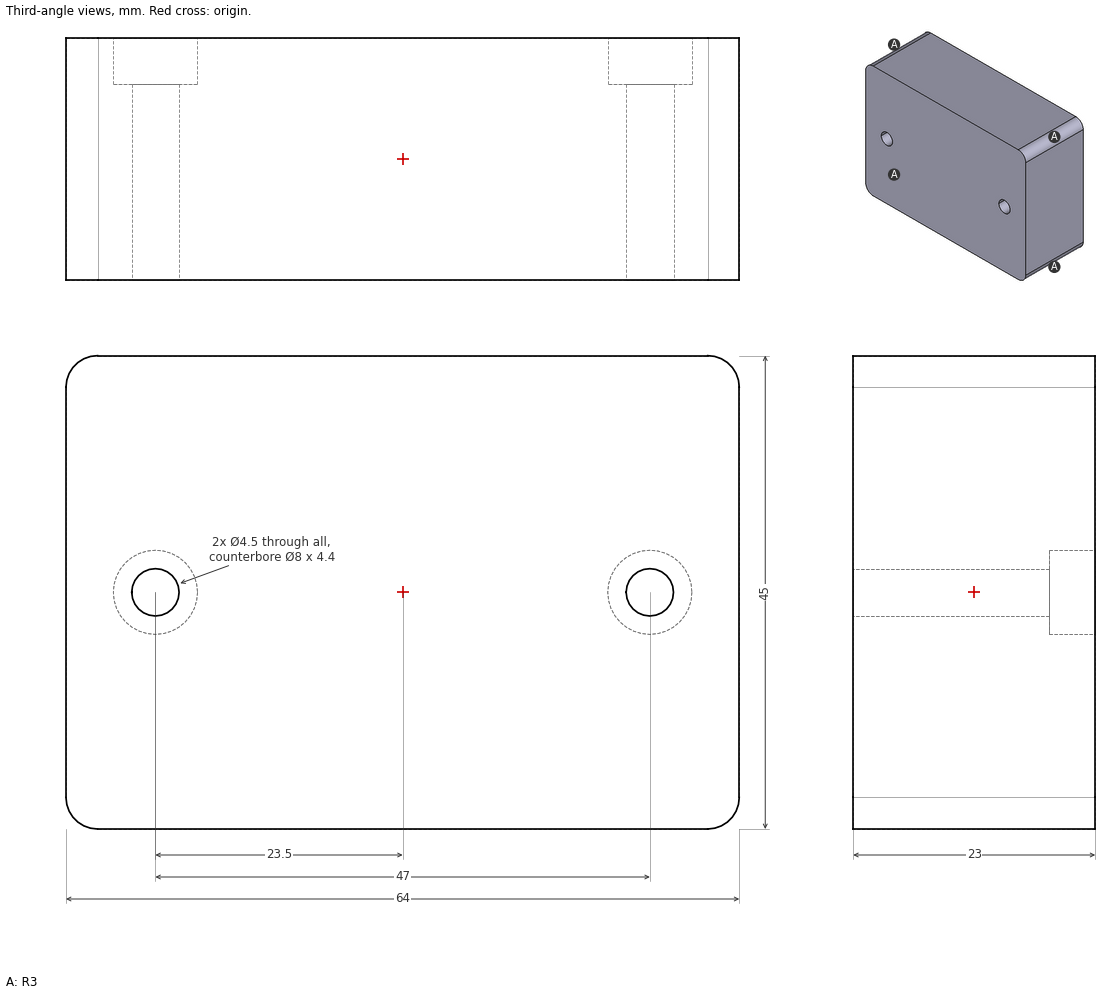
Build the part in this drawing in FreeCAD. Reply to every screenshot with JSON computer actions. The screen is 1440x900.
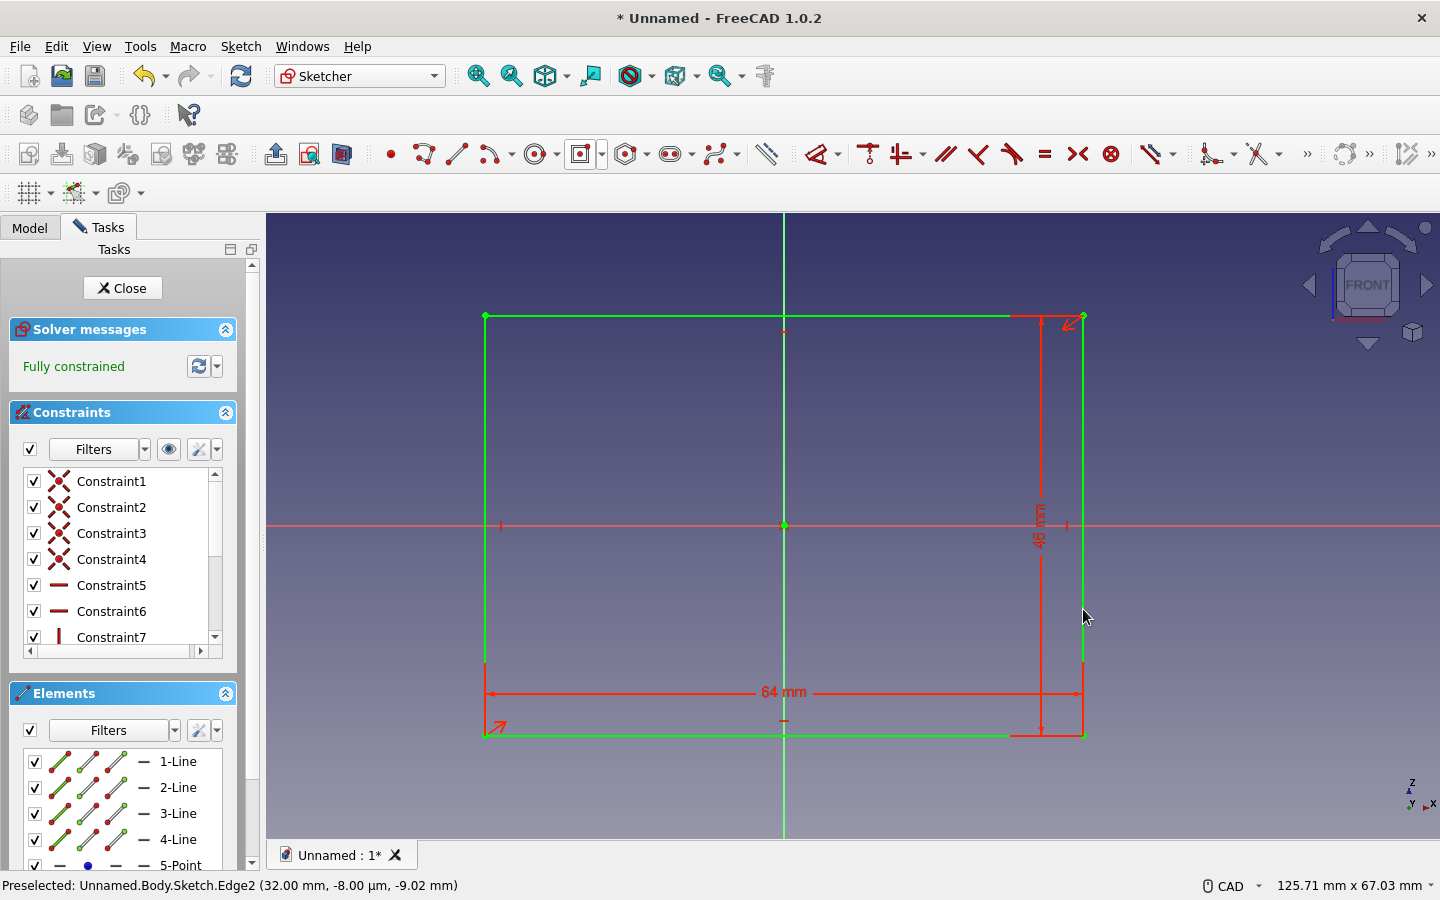
{"action": "left_click", "coordinate": [123, 288]}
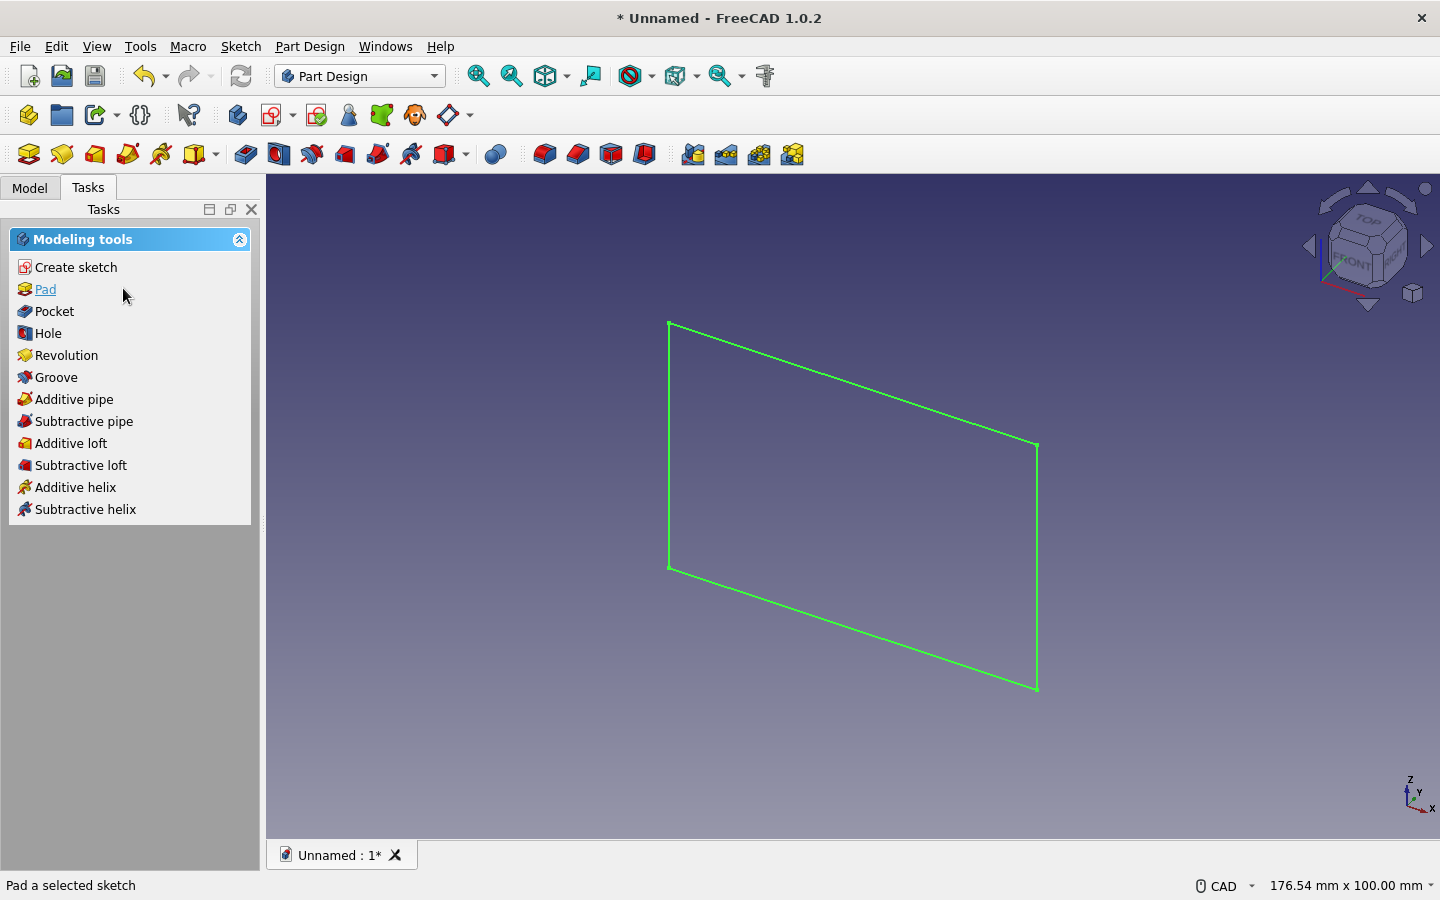
{"action": "left_click", "coordinate": [29, 154]}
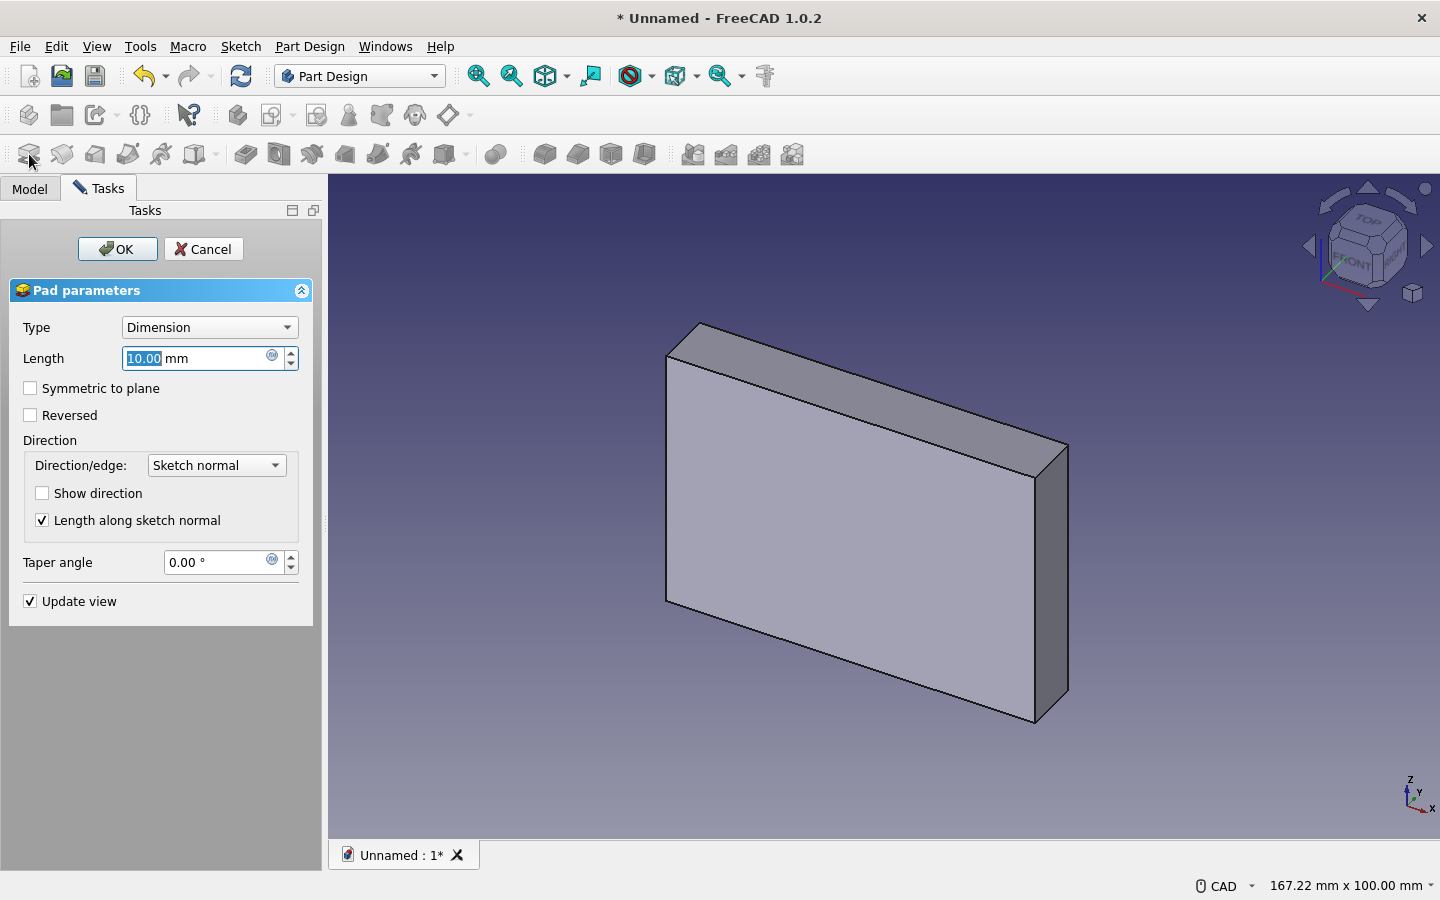
{"action": "type", "text": "23"}
{"action": "key", "text": "Tab"}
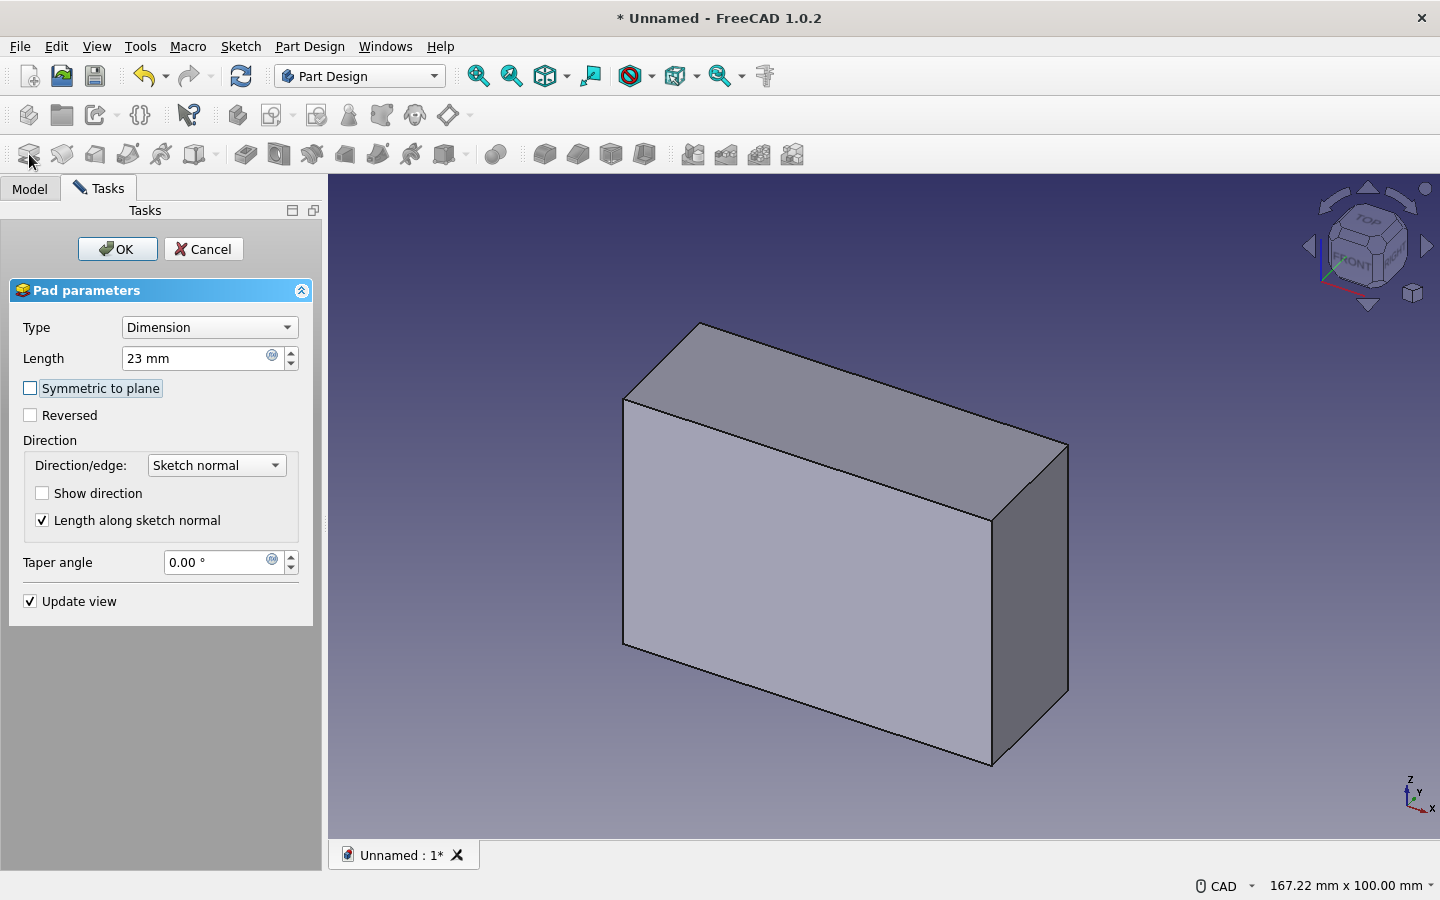
{"action": "left_click", "coordinate": [31, 388]}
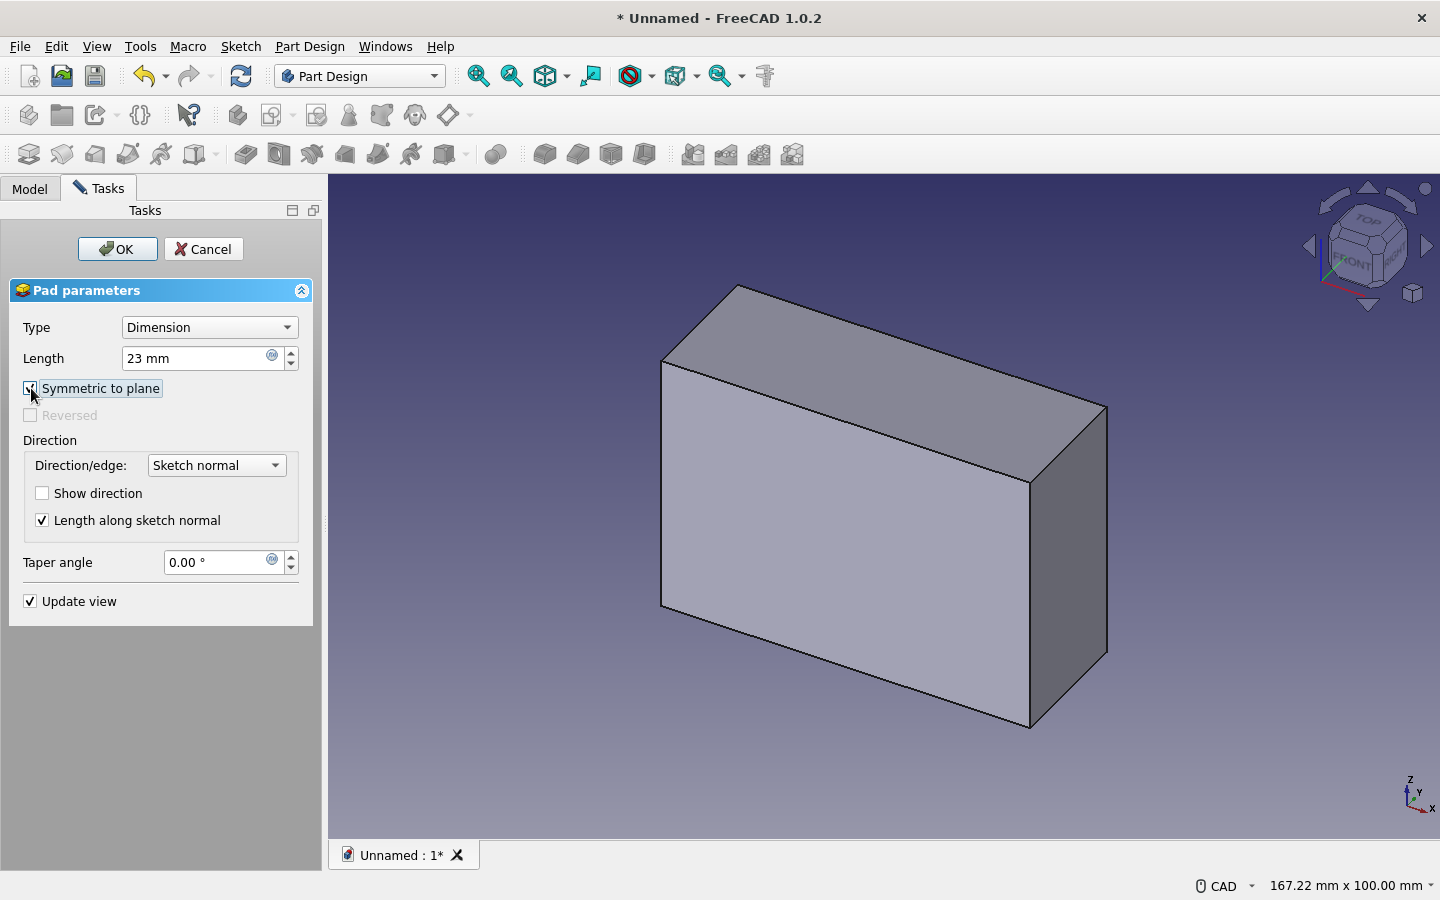
{"action": "left_click", "coordinate": [118, 249]}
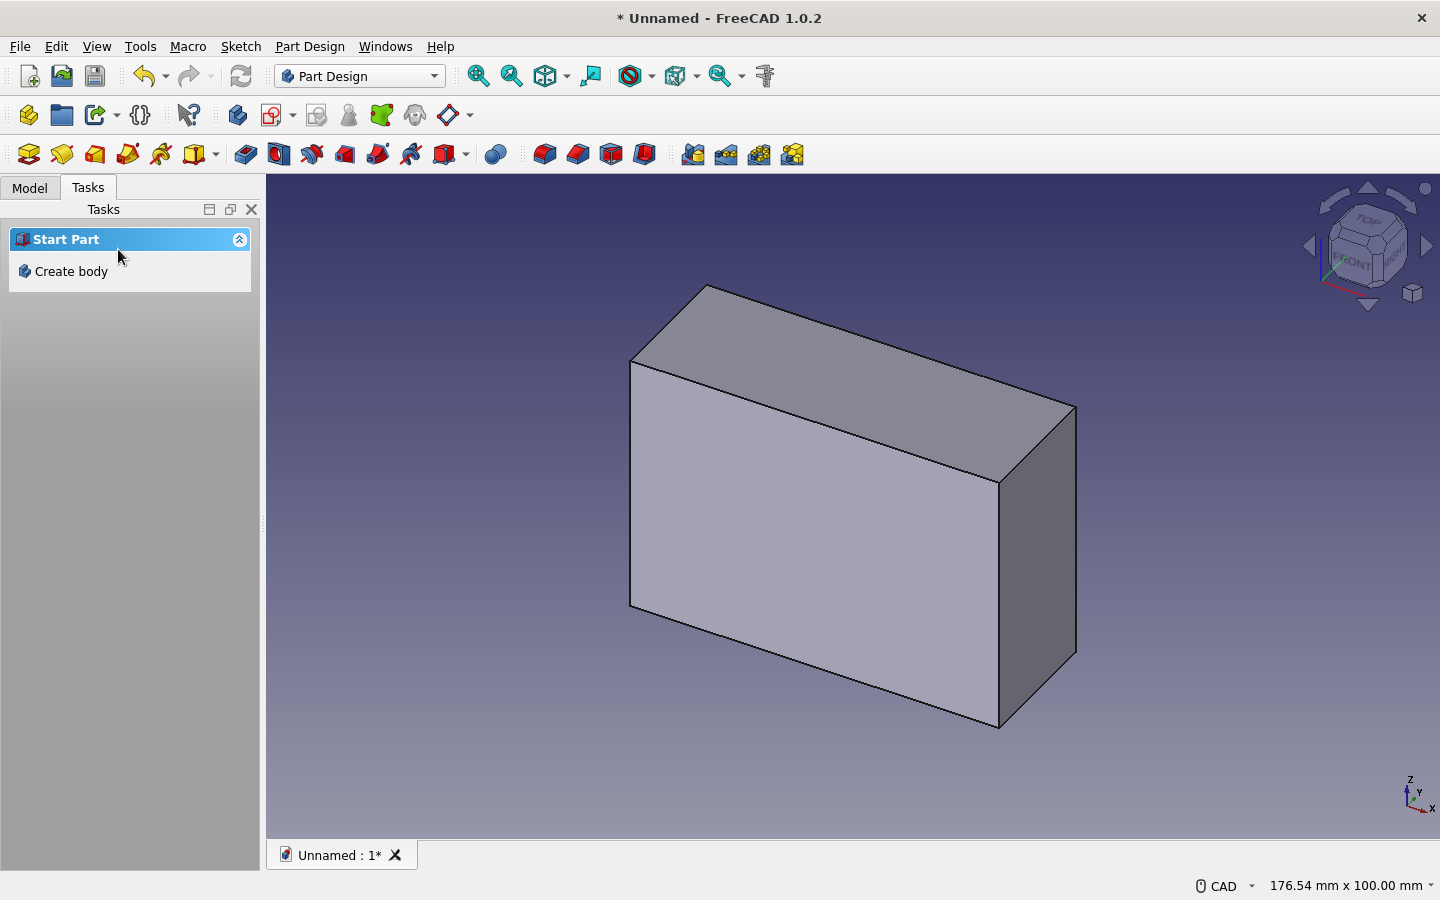
{"action": "key", "text": "4"}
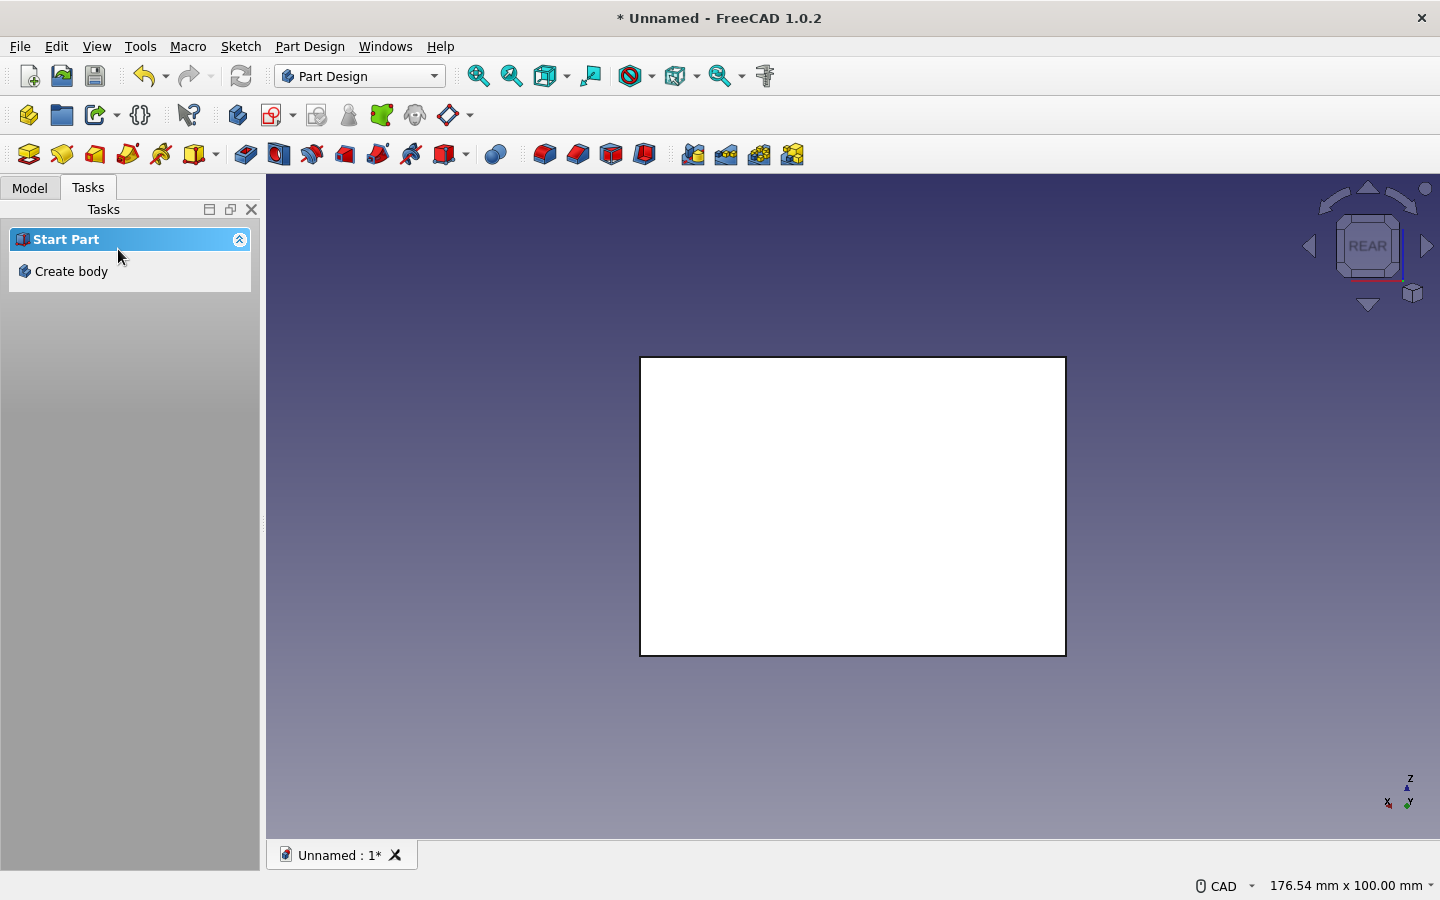
{"action": "left_click", "coordinate": [479, 76]}